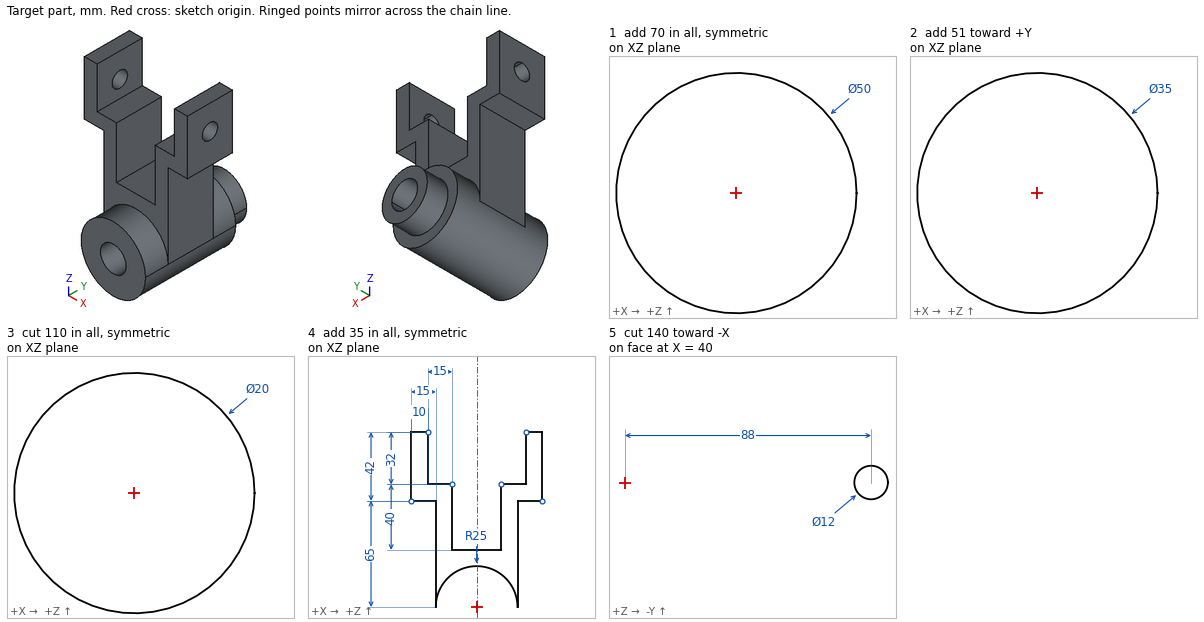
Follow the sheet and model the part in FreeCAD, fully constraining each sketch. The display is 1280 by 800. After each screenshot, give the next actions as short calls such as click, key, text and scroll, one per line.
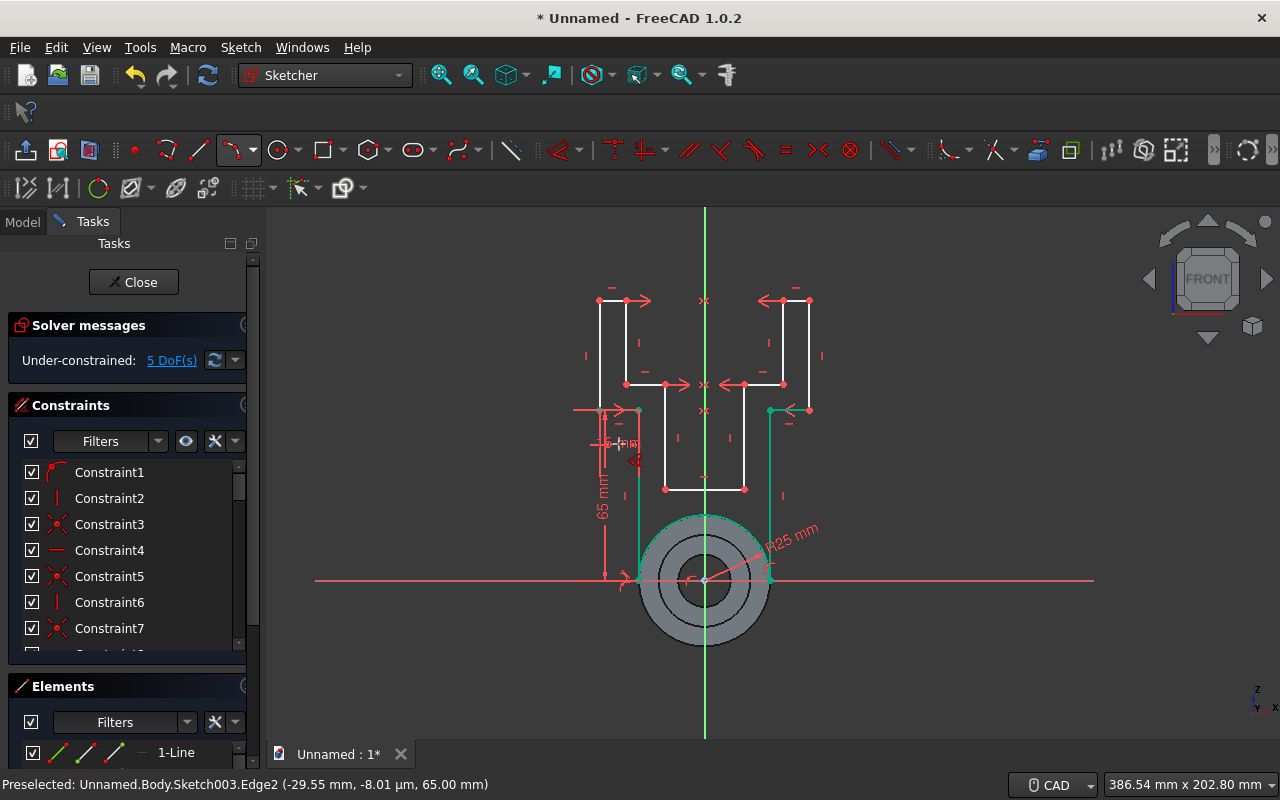
click(600, 378)
click(566, 356)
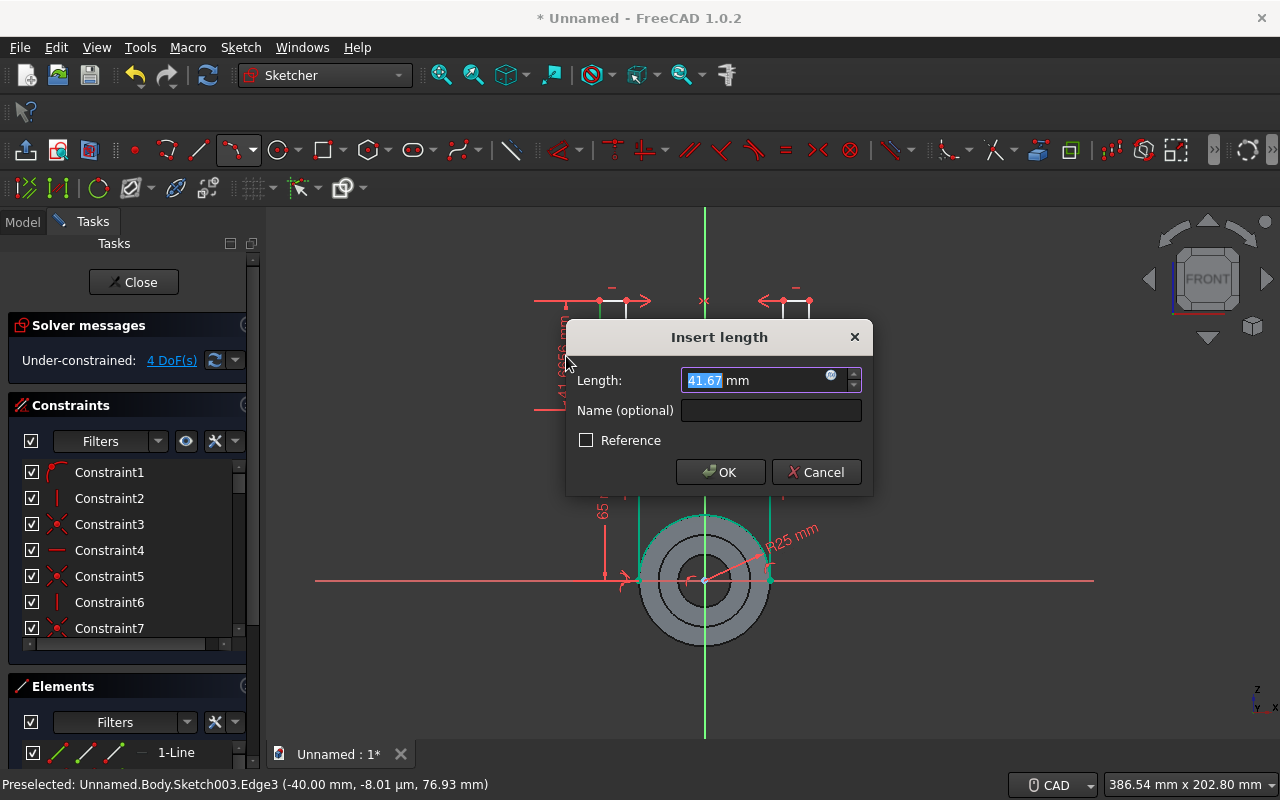
text(42)
key(Return)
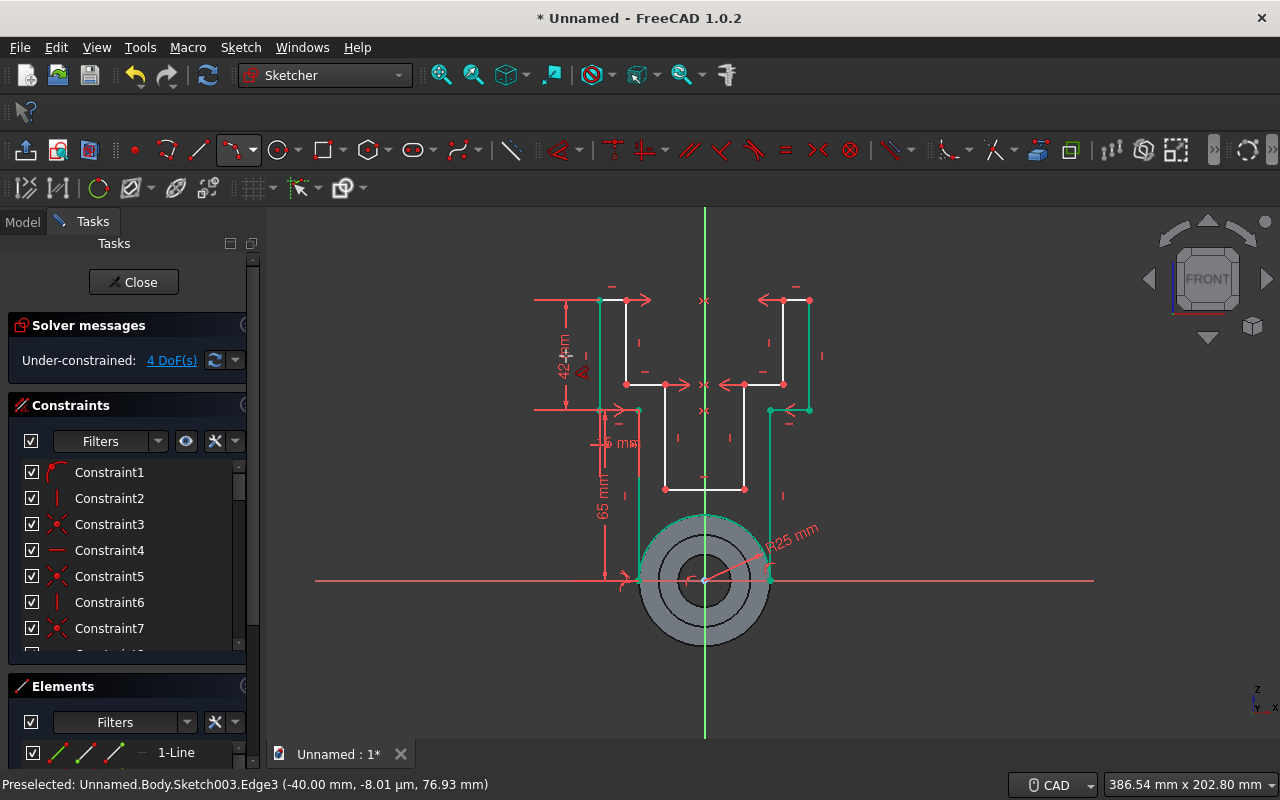
scroll(610, 300, up, 3)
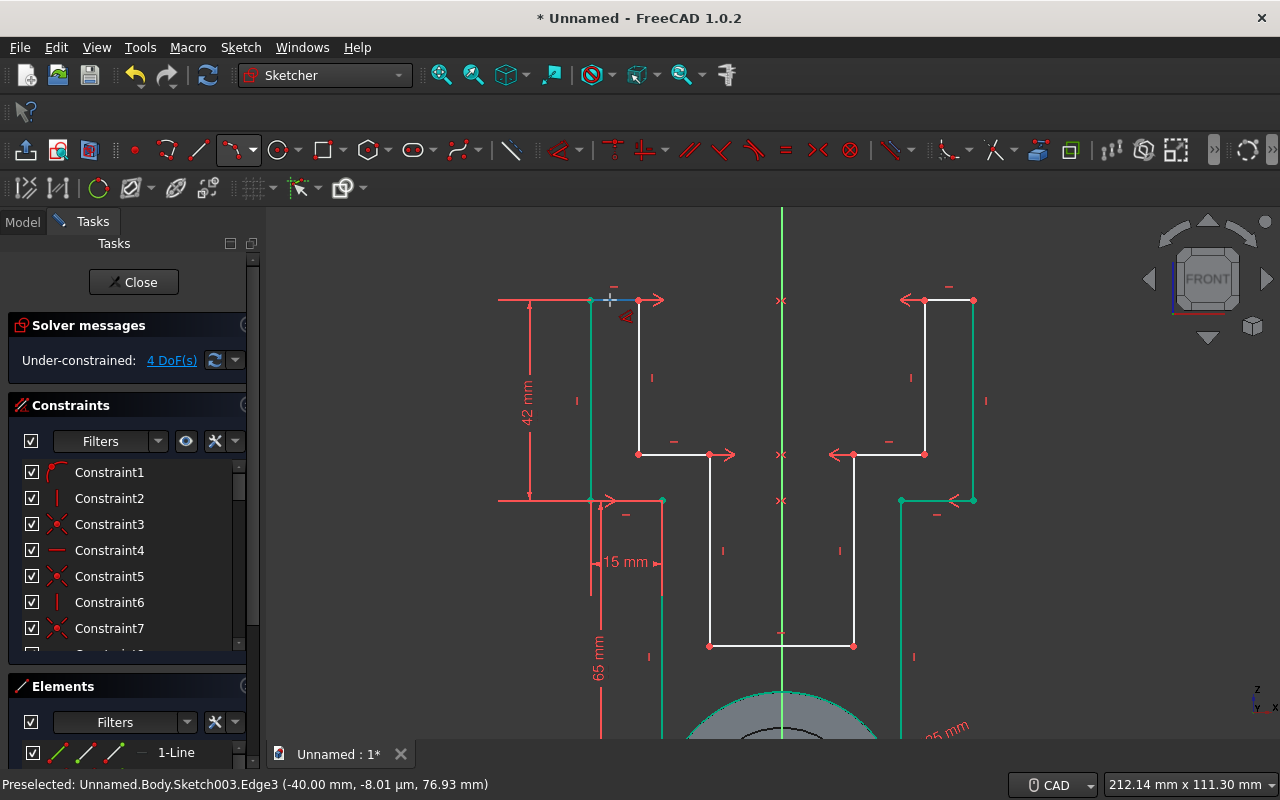
click(610, 300)
click(615, 266)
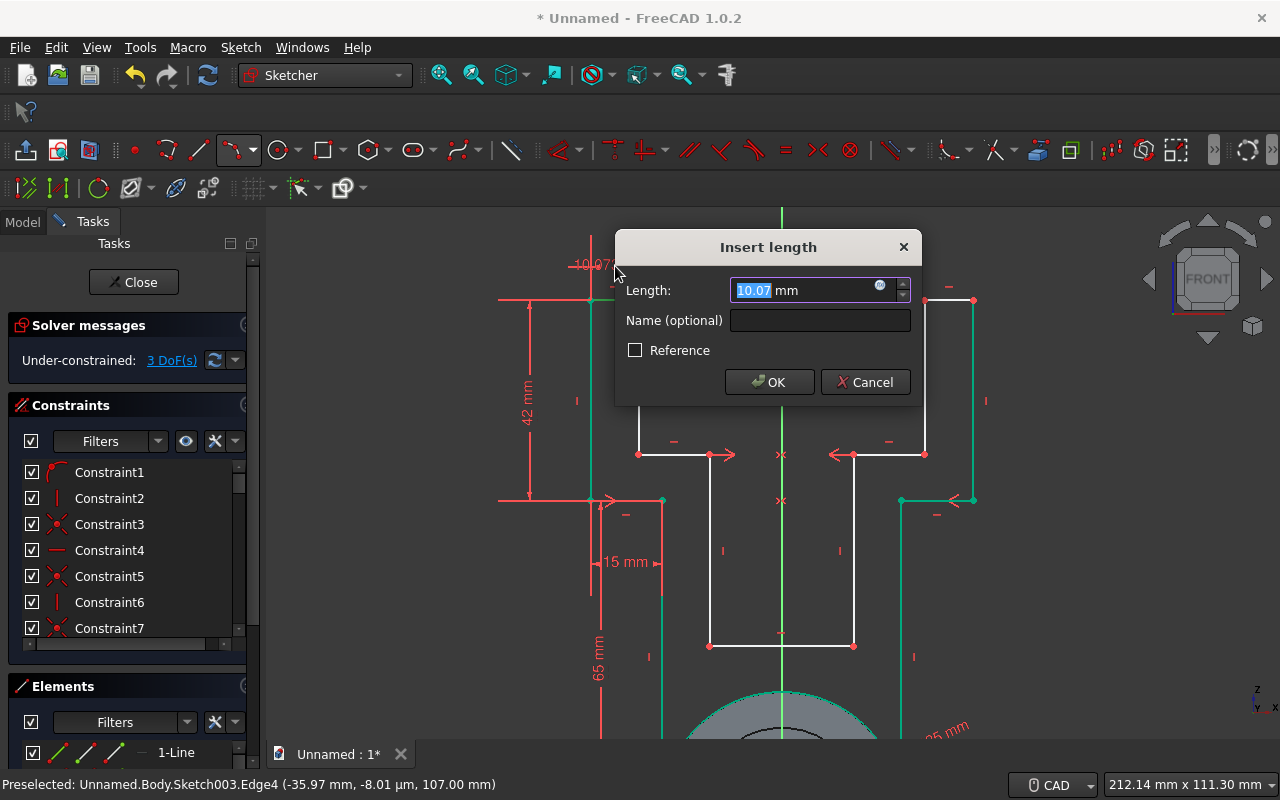
text(10)
key(Return)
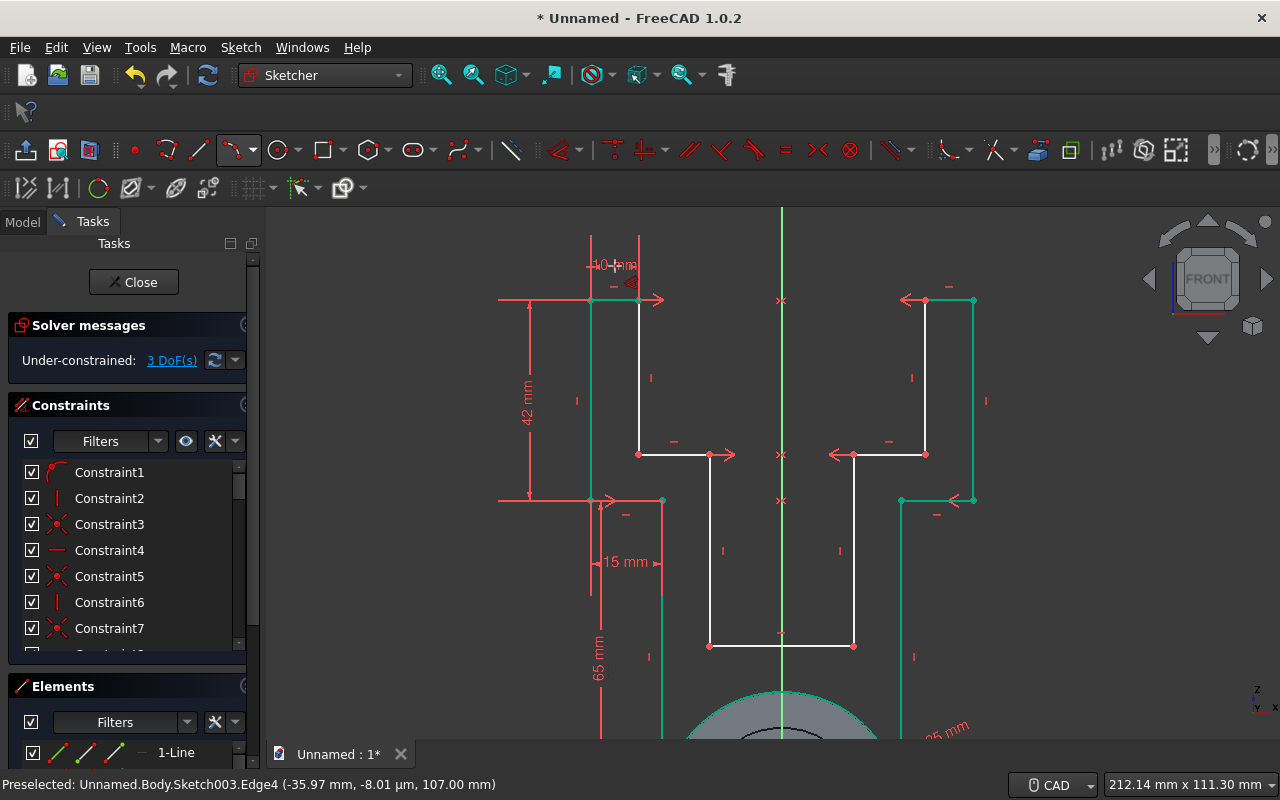
click(639, 346)
click(605, 377)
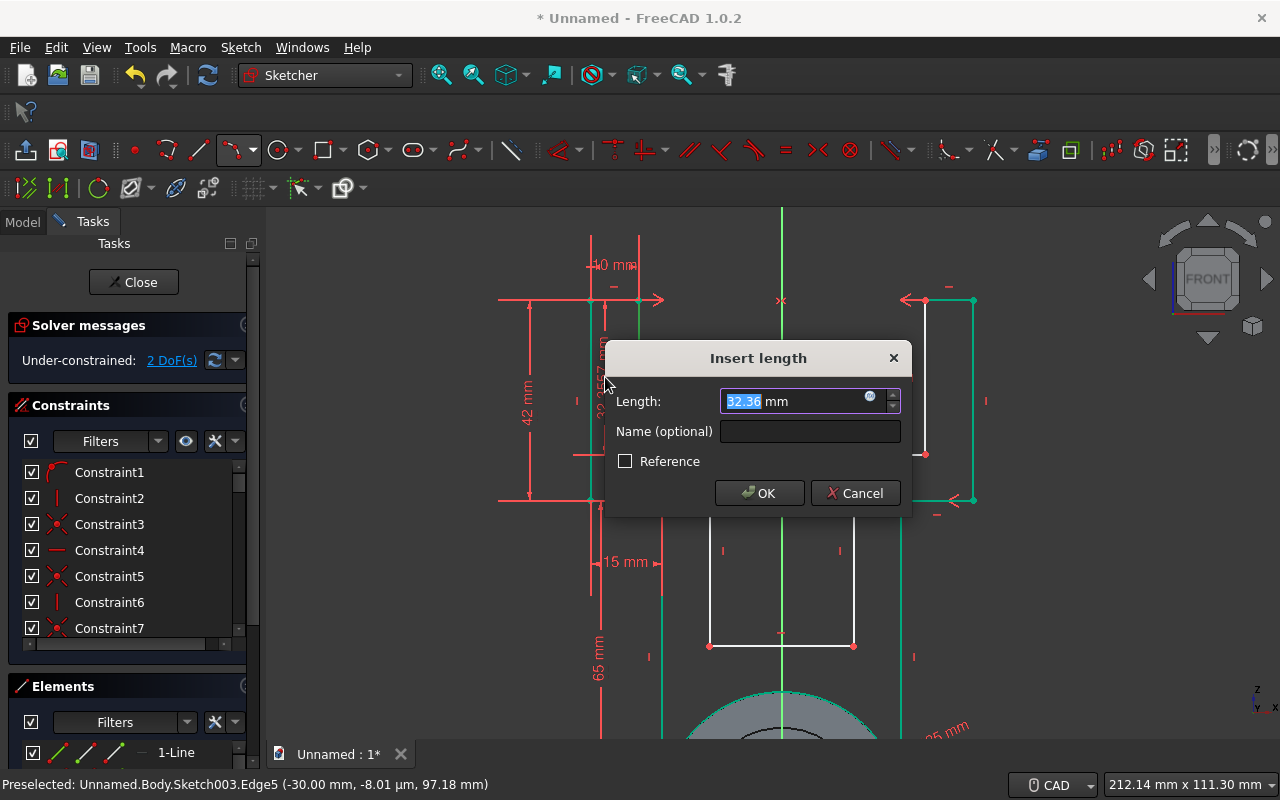
text(32)
key(Return)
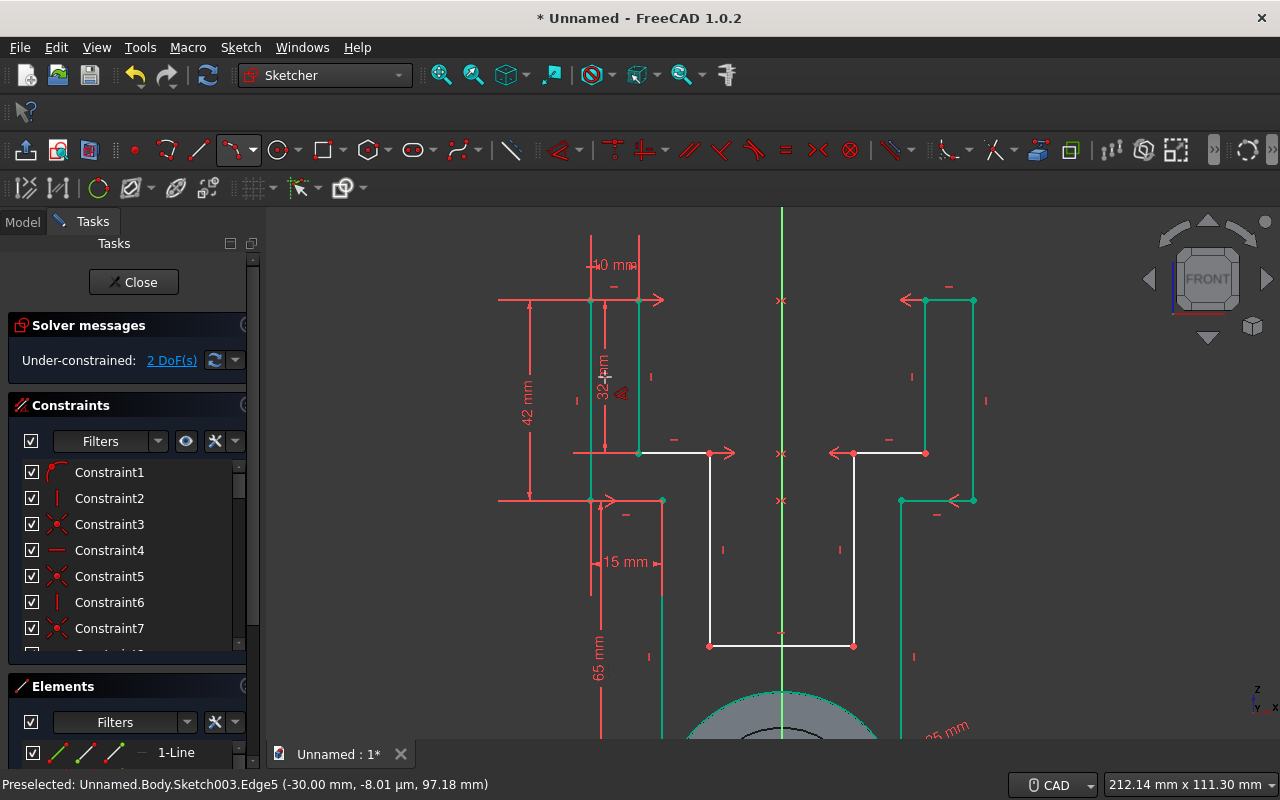
click(660, 453)
click(674, 419)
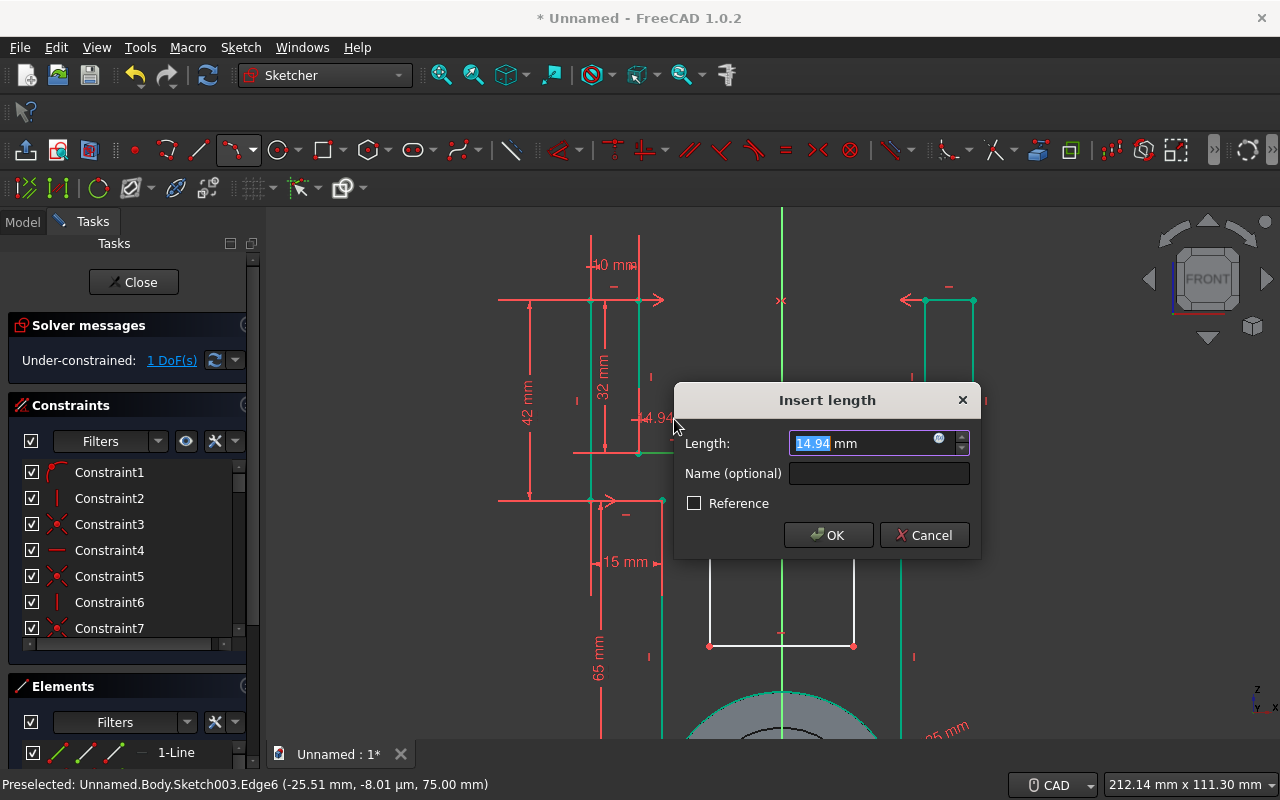
text(15)
key(Return)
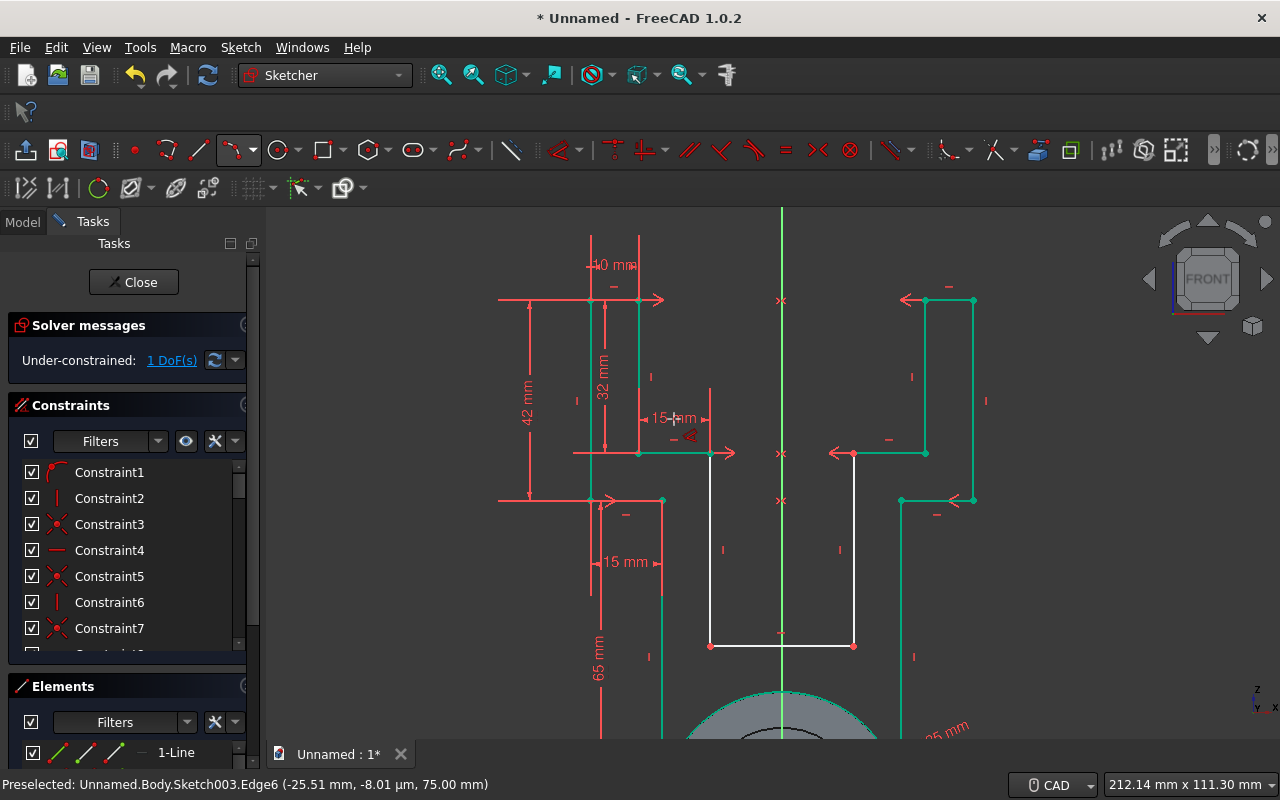
click(710, 511)
click(676, 505)